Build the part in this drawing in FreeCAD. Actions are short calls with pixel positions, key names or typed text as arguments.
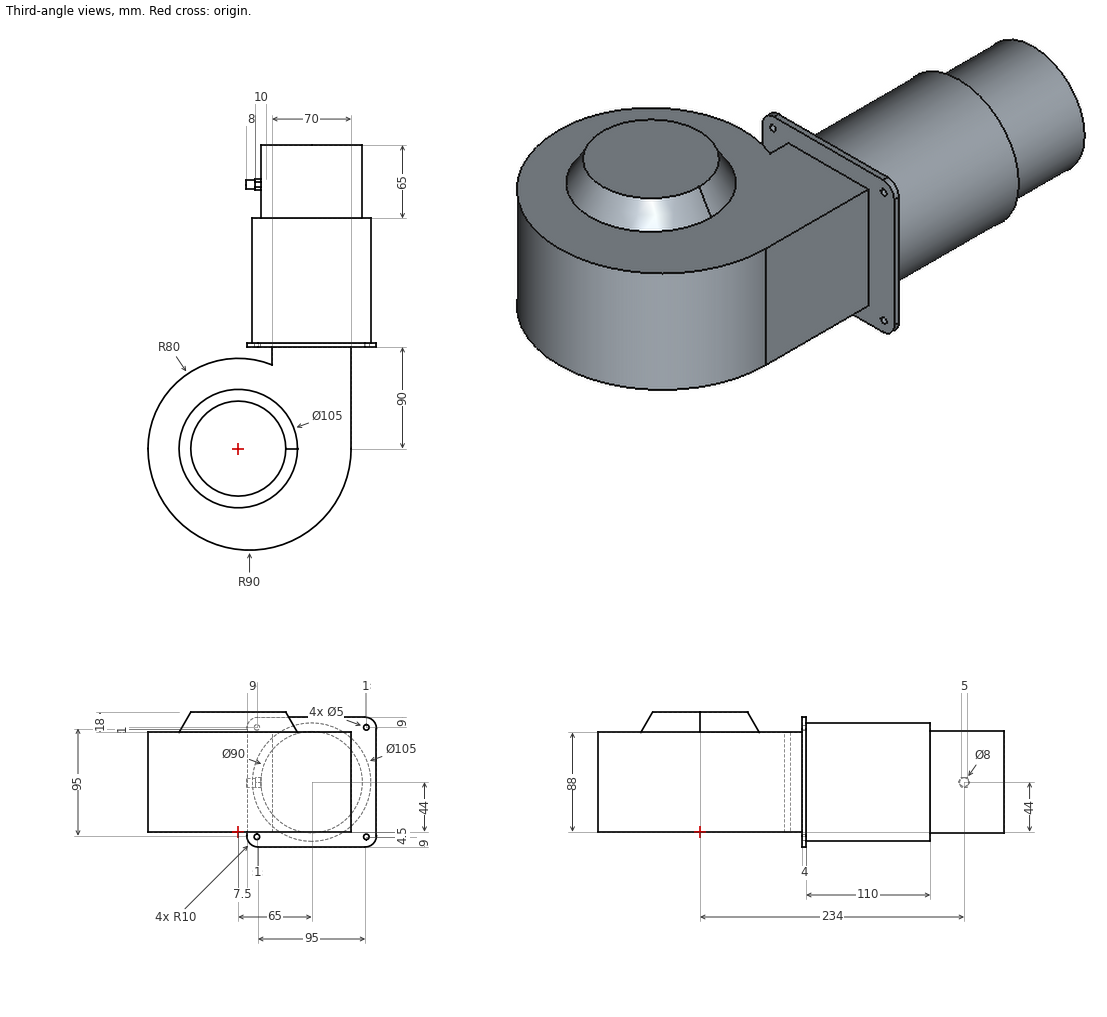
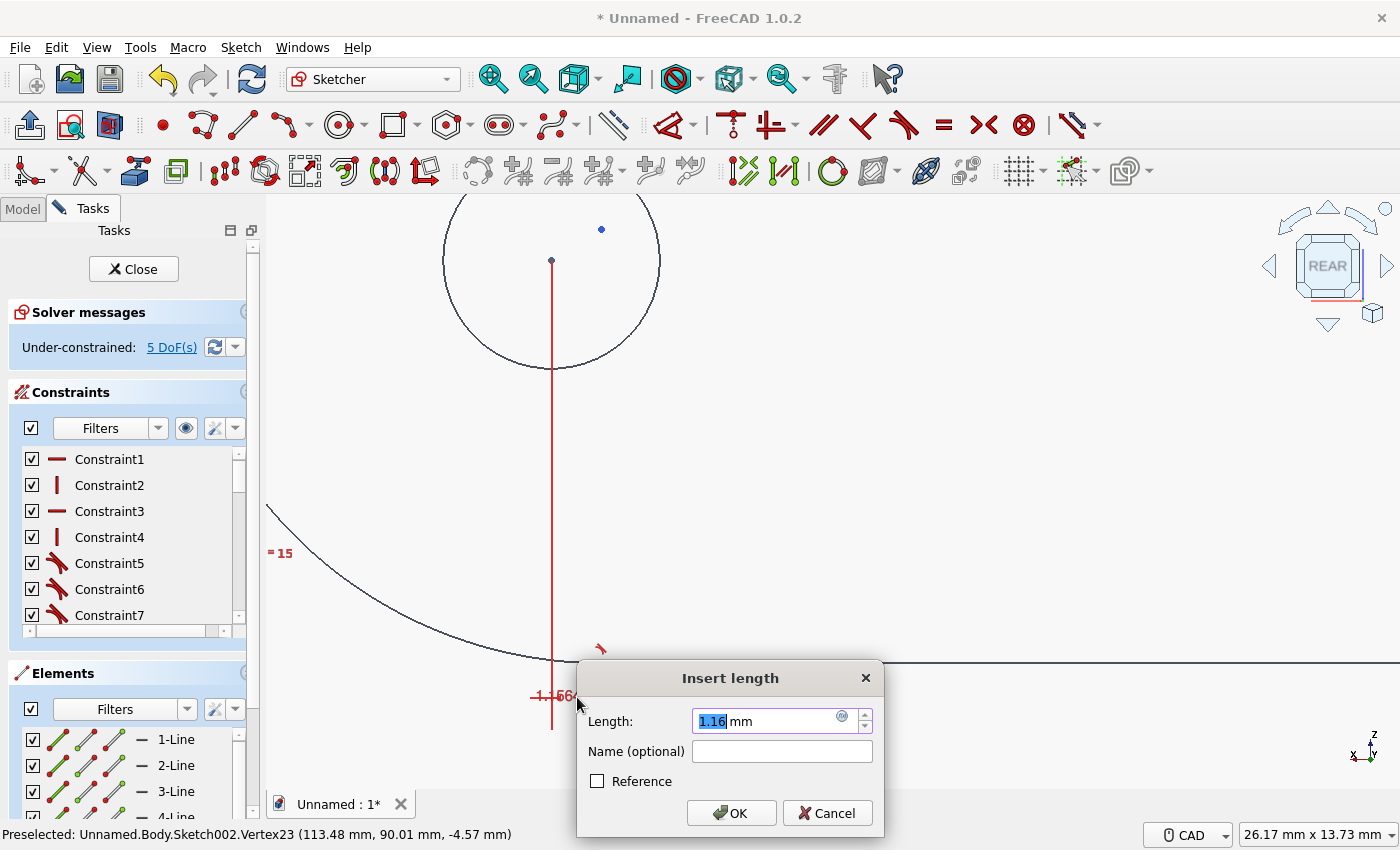
text(1)
key(Return)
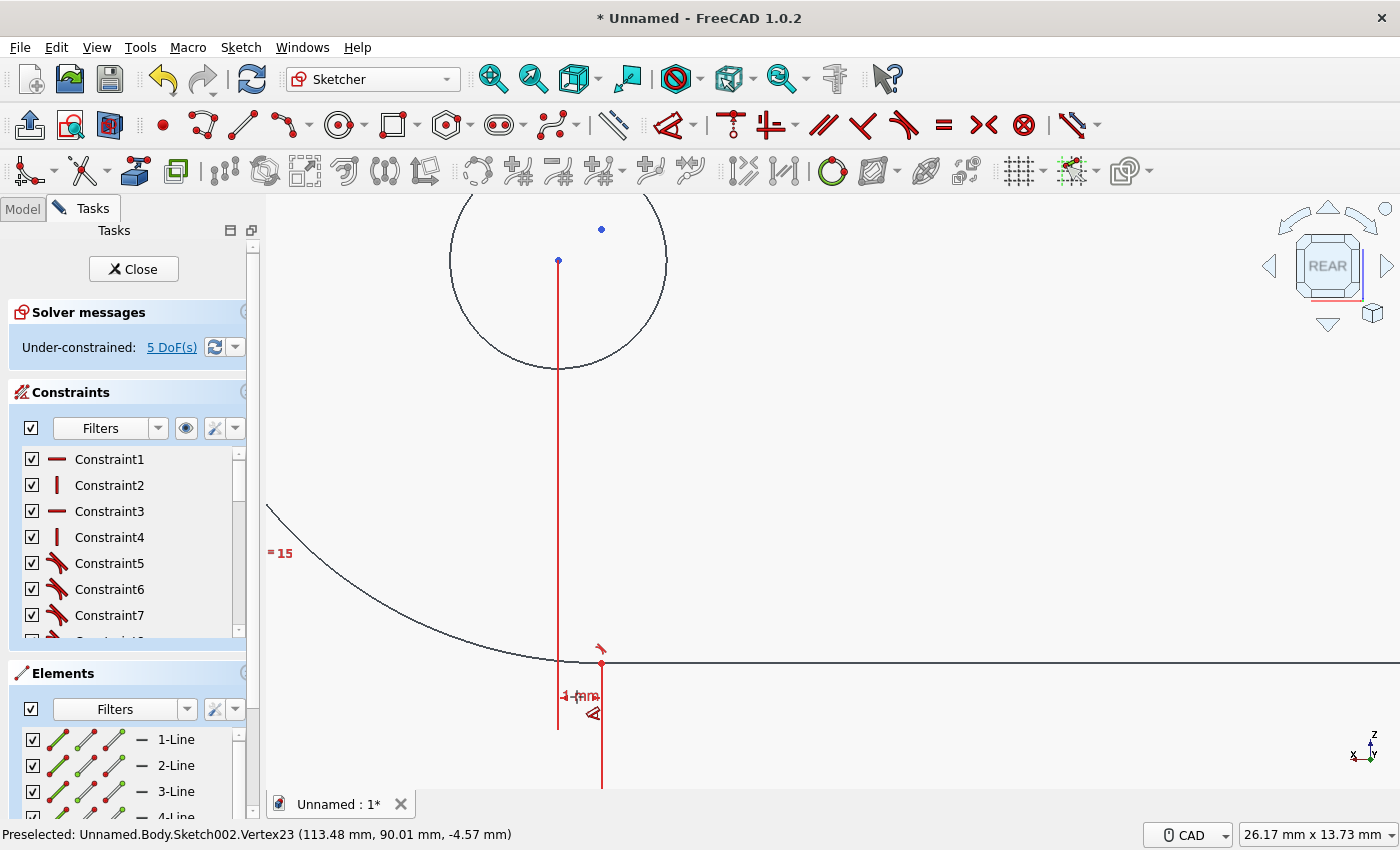
scroll(600, 679, down, 13)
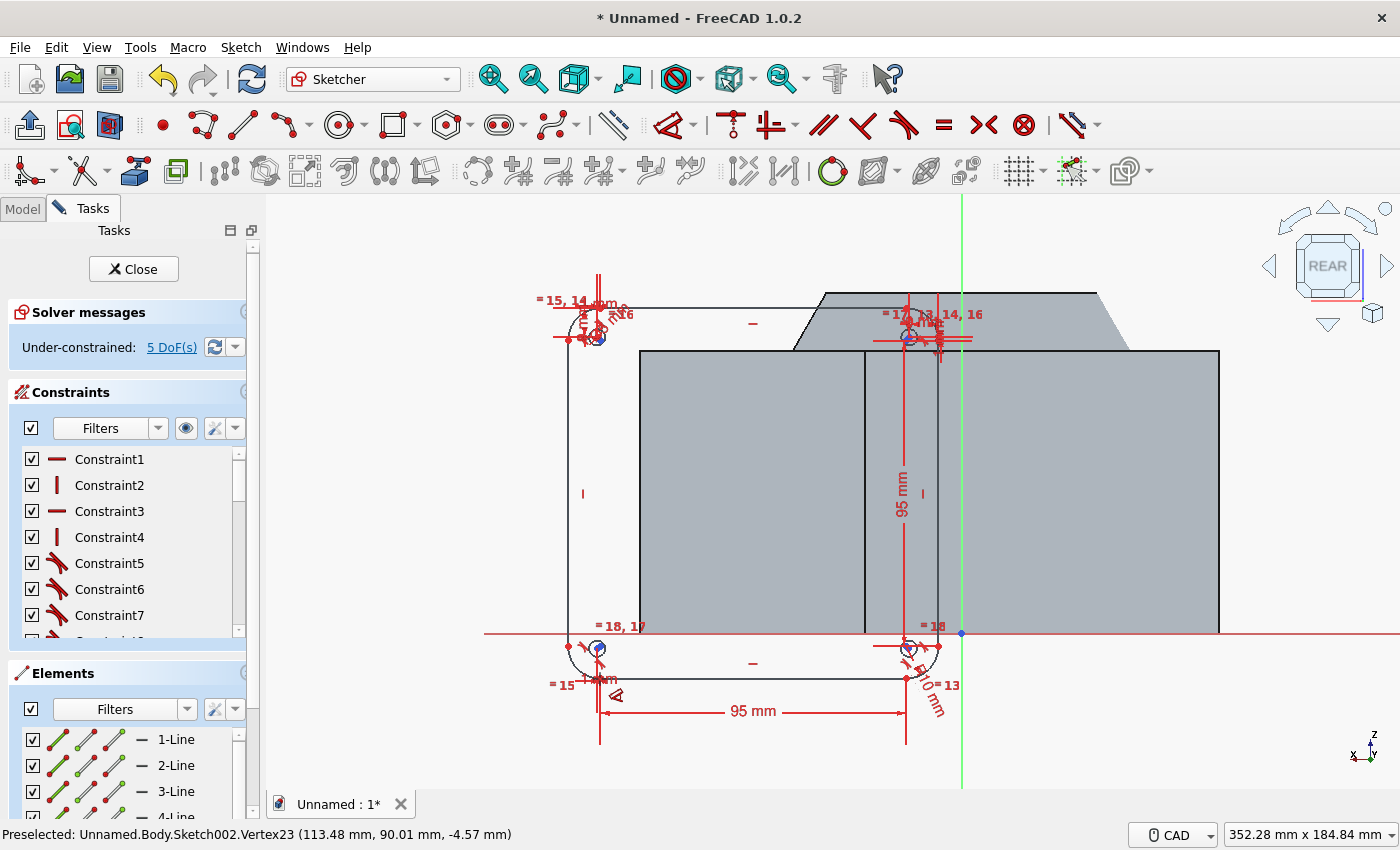
scroll(600, 679, up, 2)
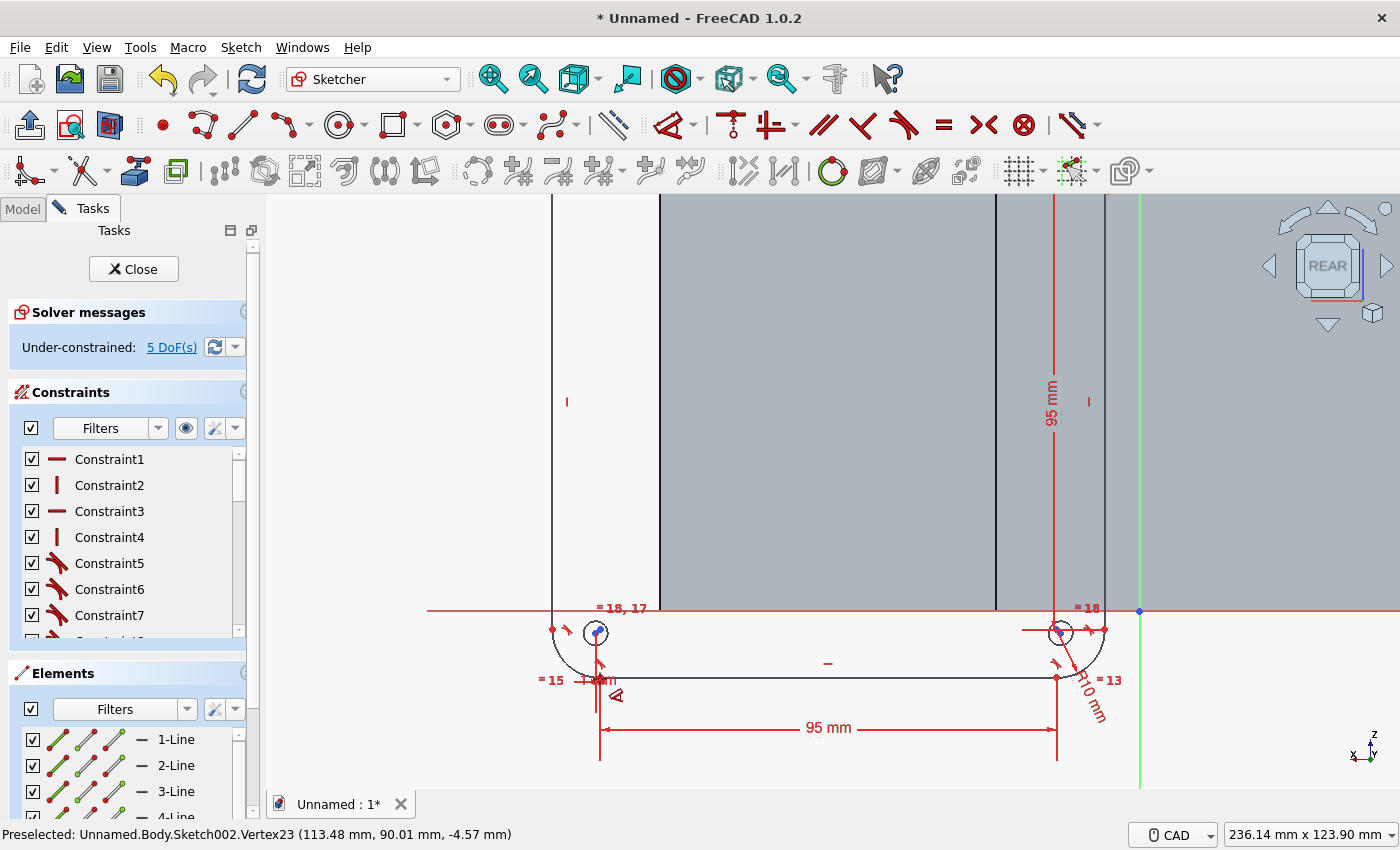
click(600, 678)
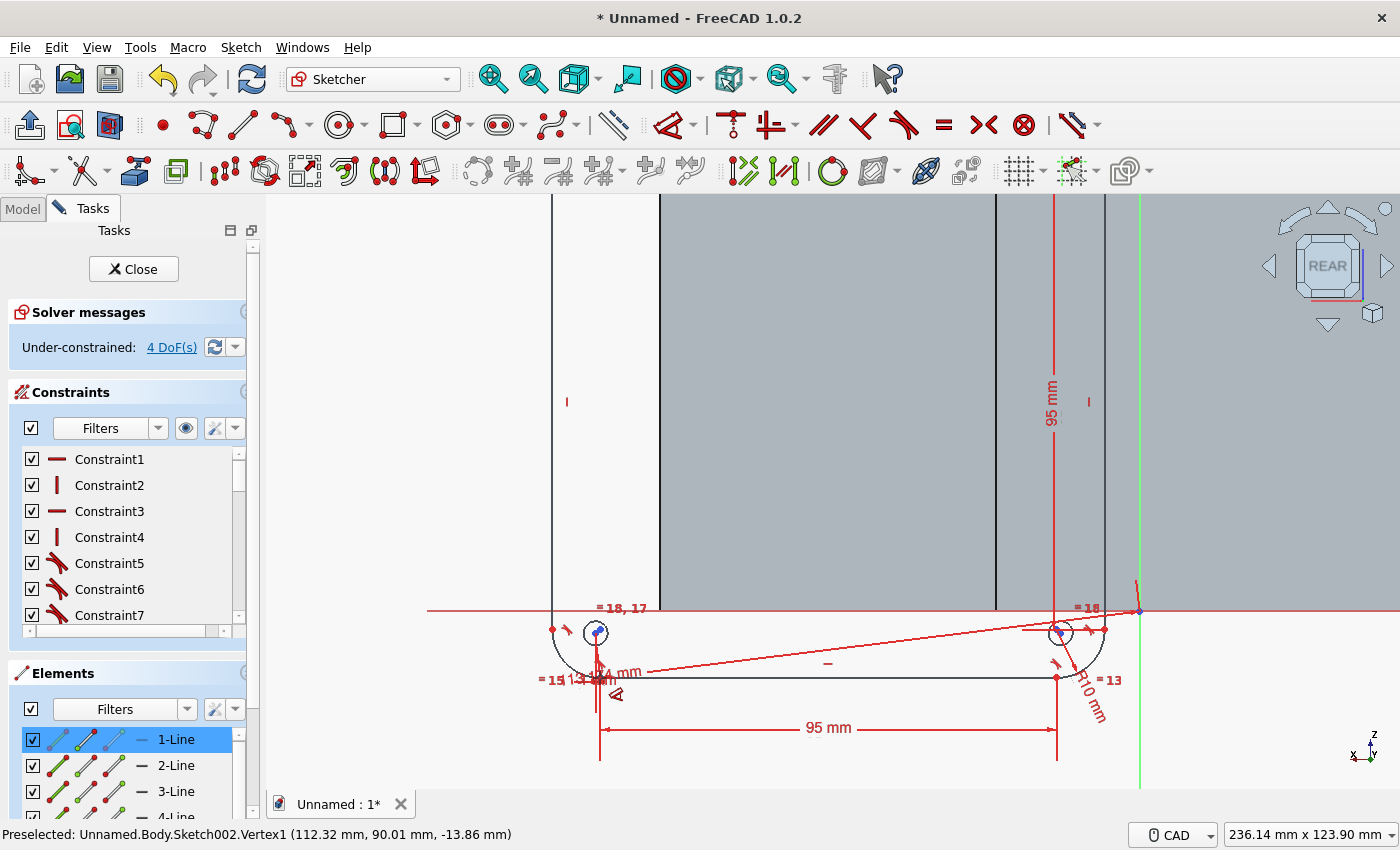
scroll(596, 633, up, 4)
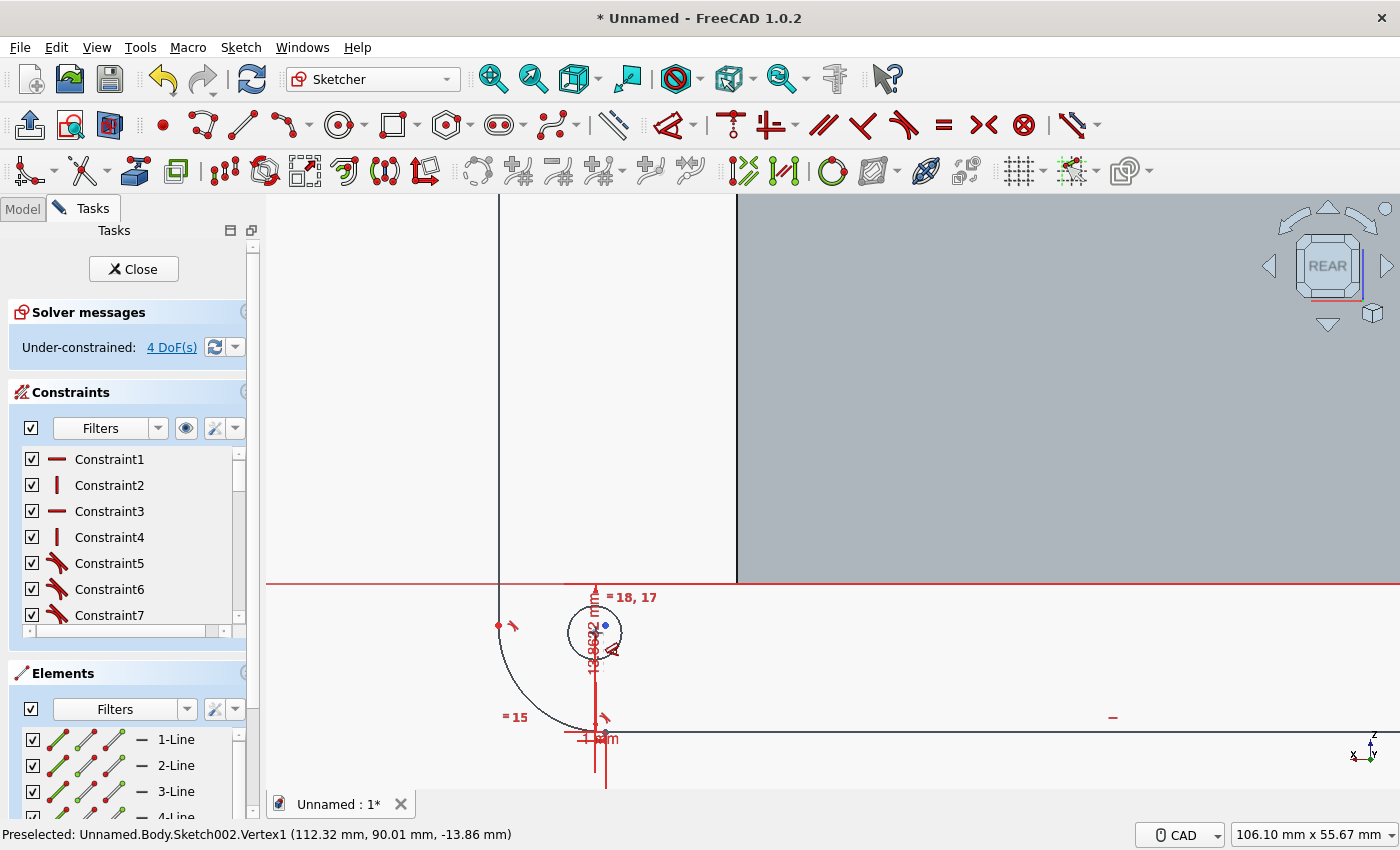
click(595, 633)
click(561, 683)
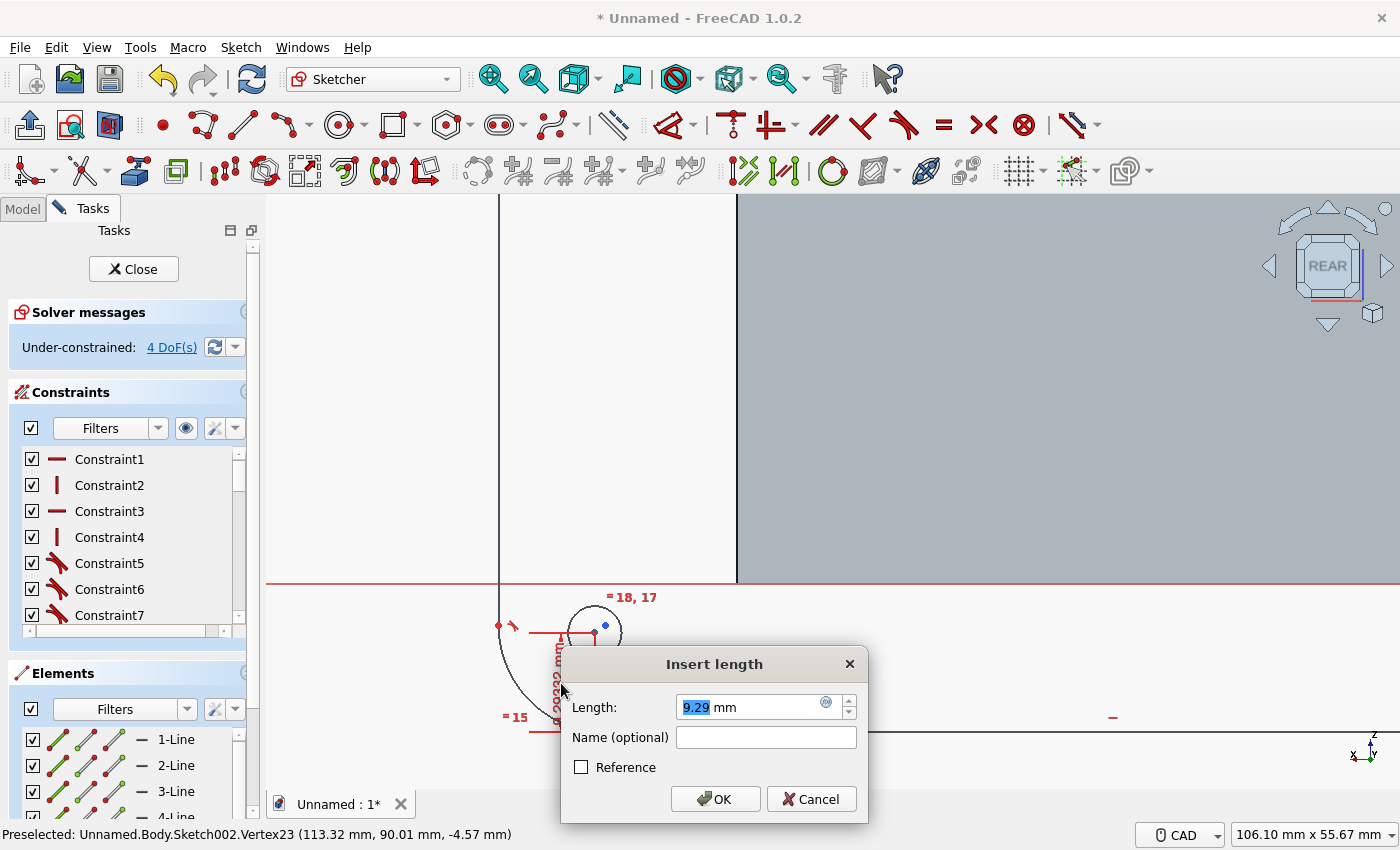
text(9)
key(Return)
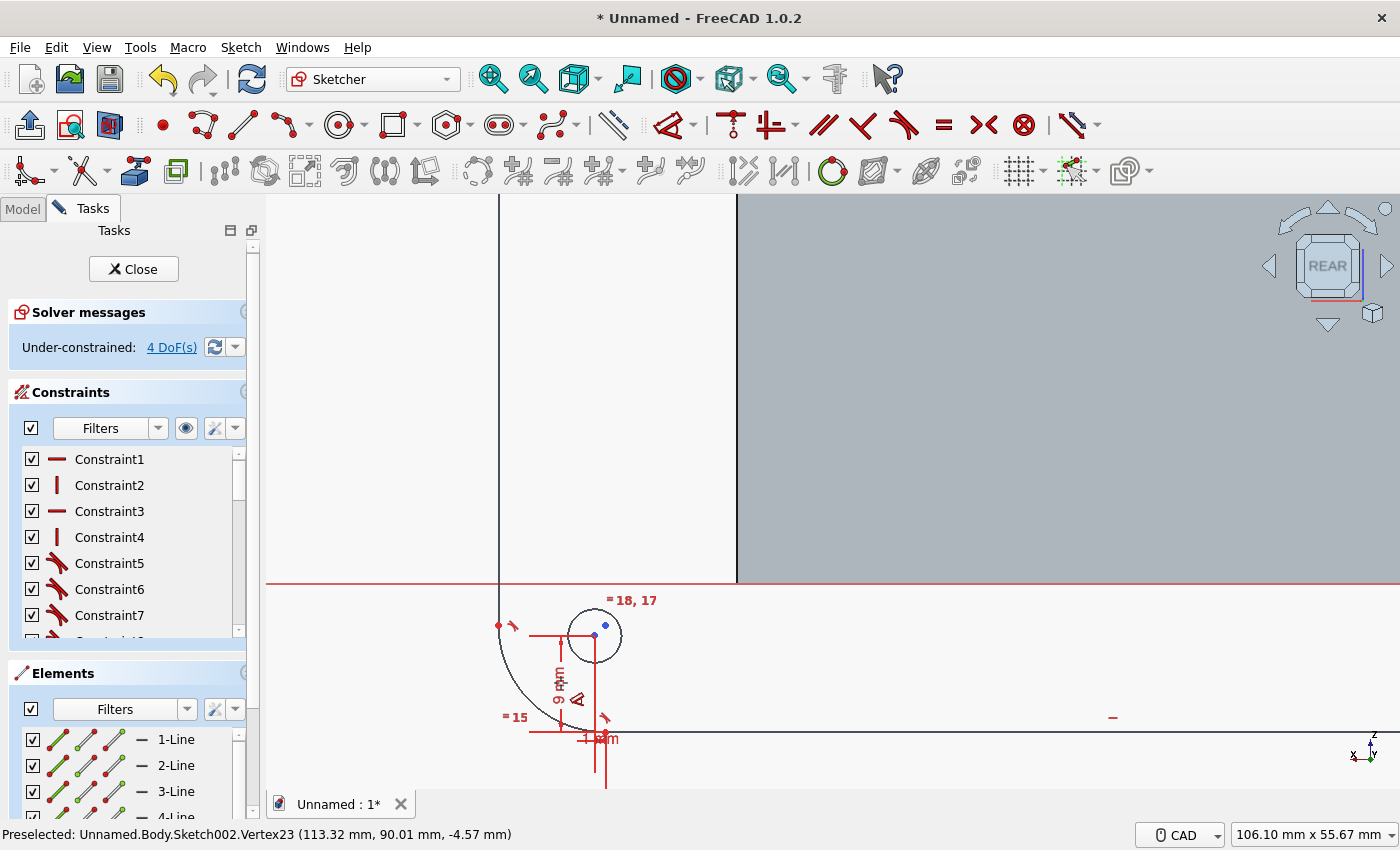
scroll(598, 654, down, 6)